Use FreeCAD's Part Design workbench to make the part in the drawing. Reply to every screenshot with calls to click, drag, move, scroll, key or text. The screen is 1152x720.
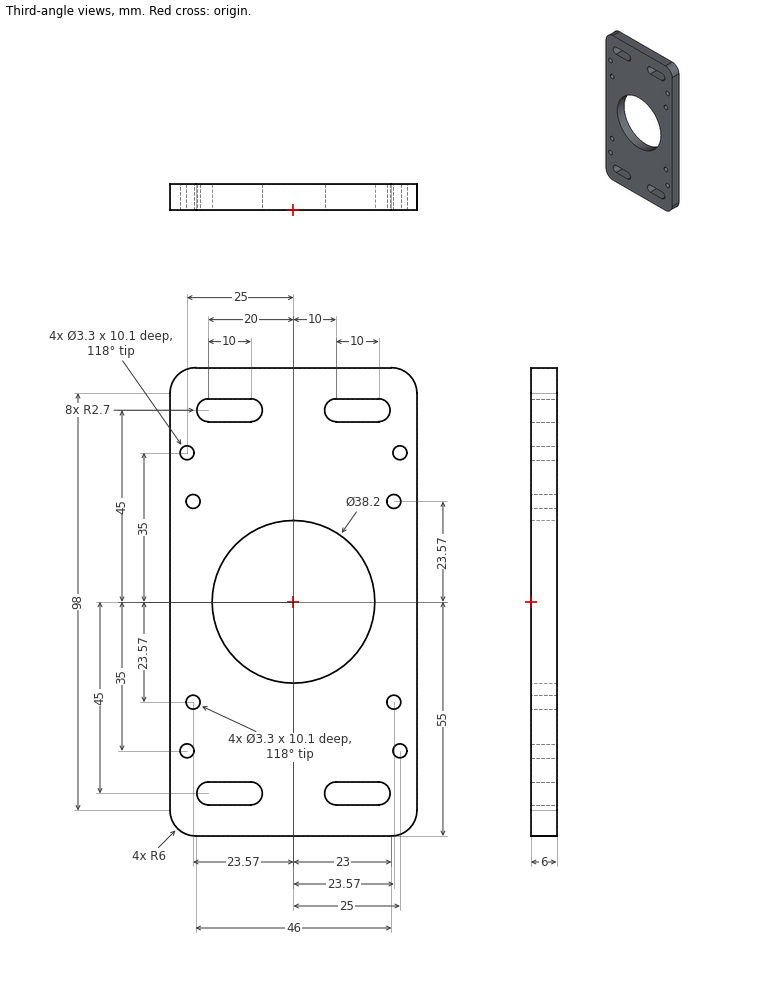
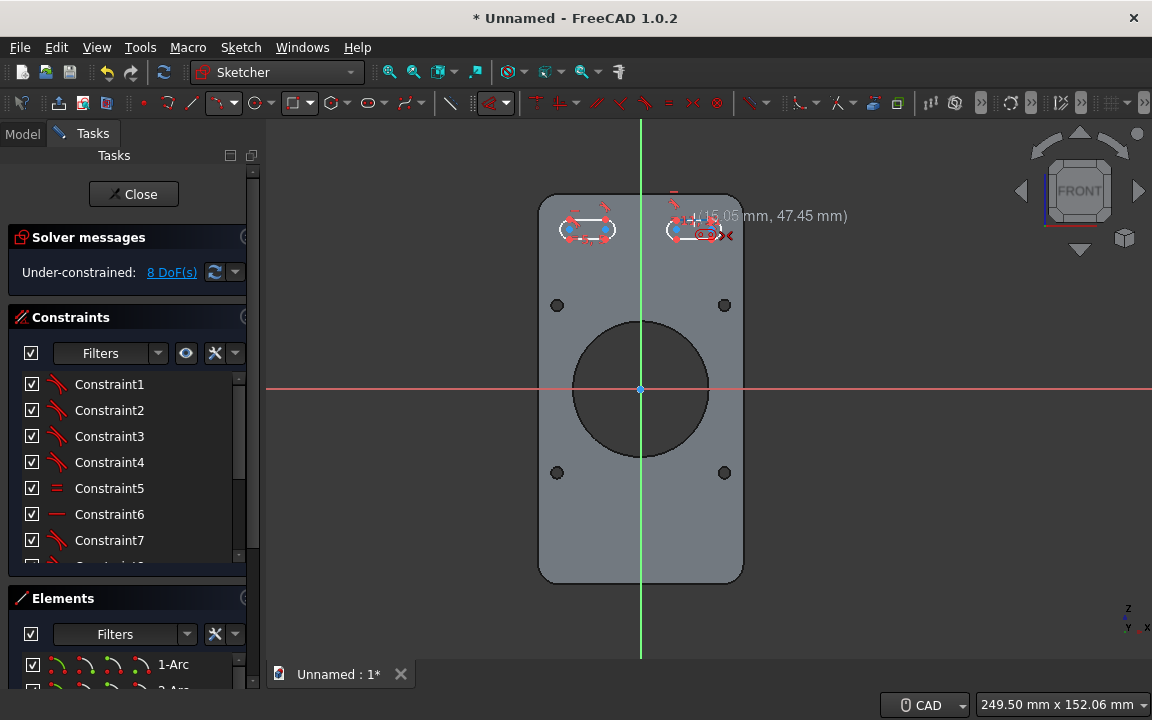
scroll(570, 549, up, 5)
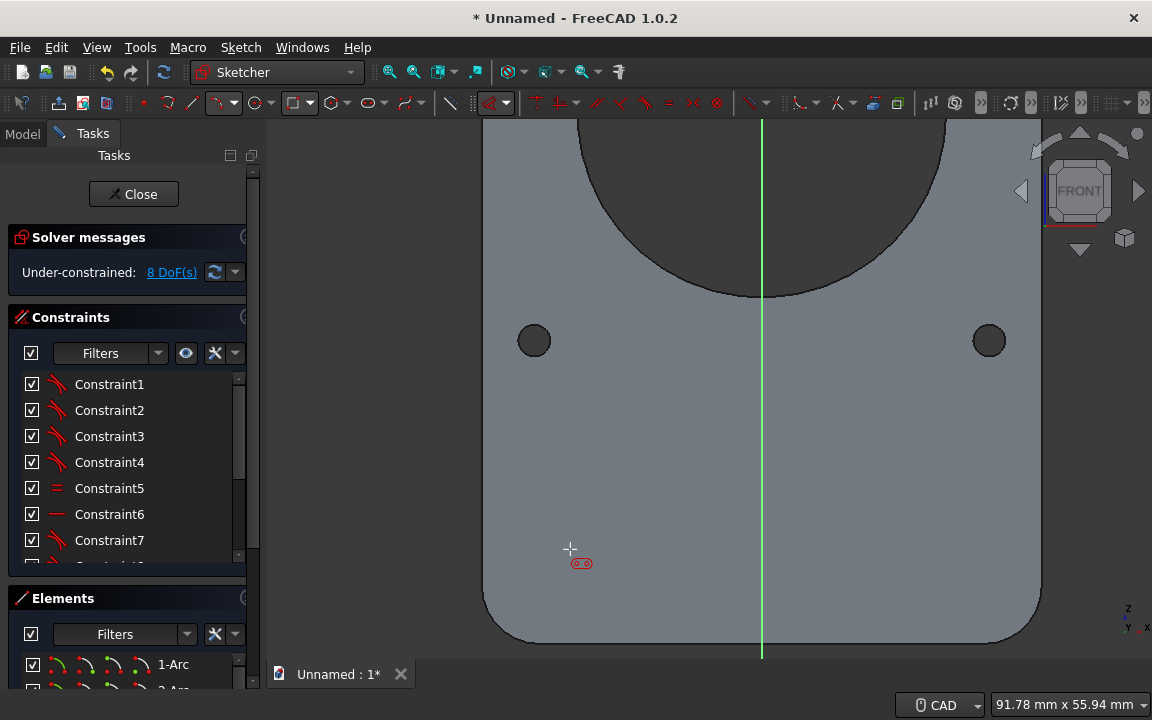
click(569, 547)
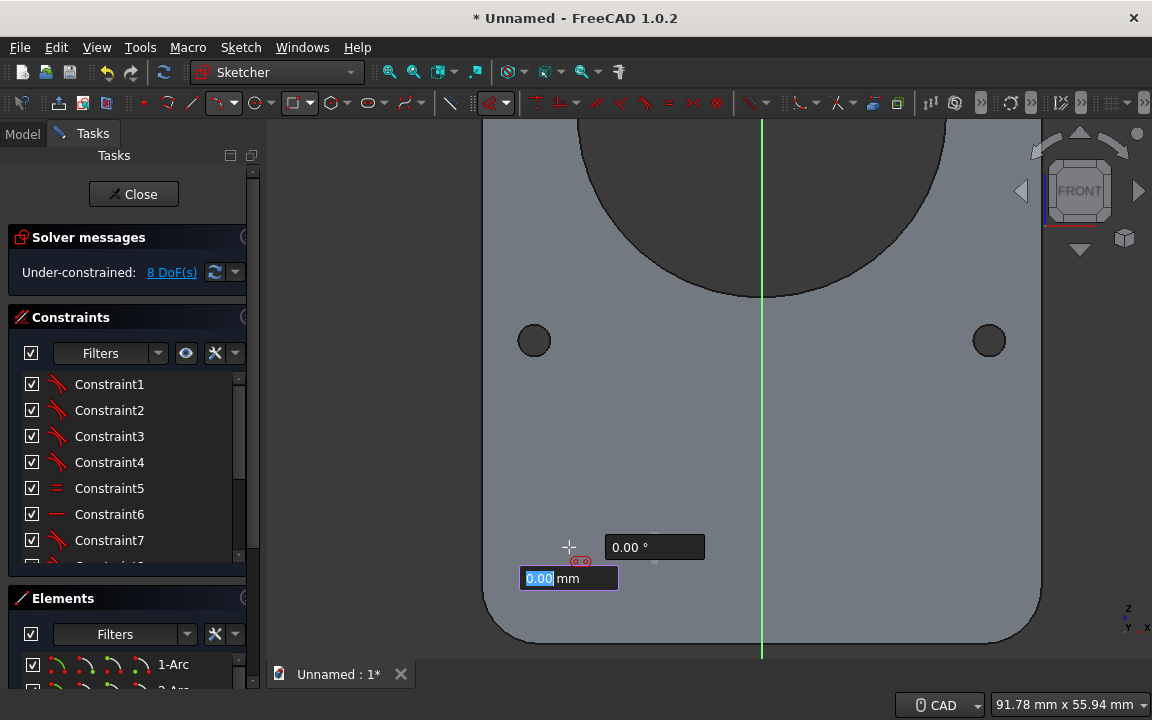
click(665, 547)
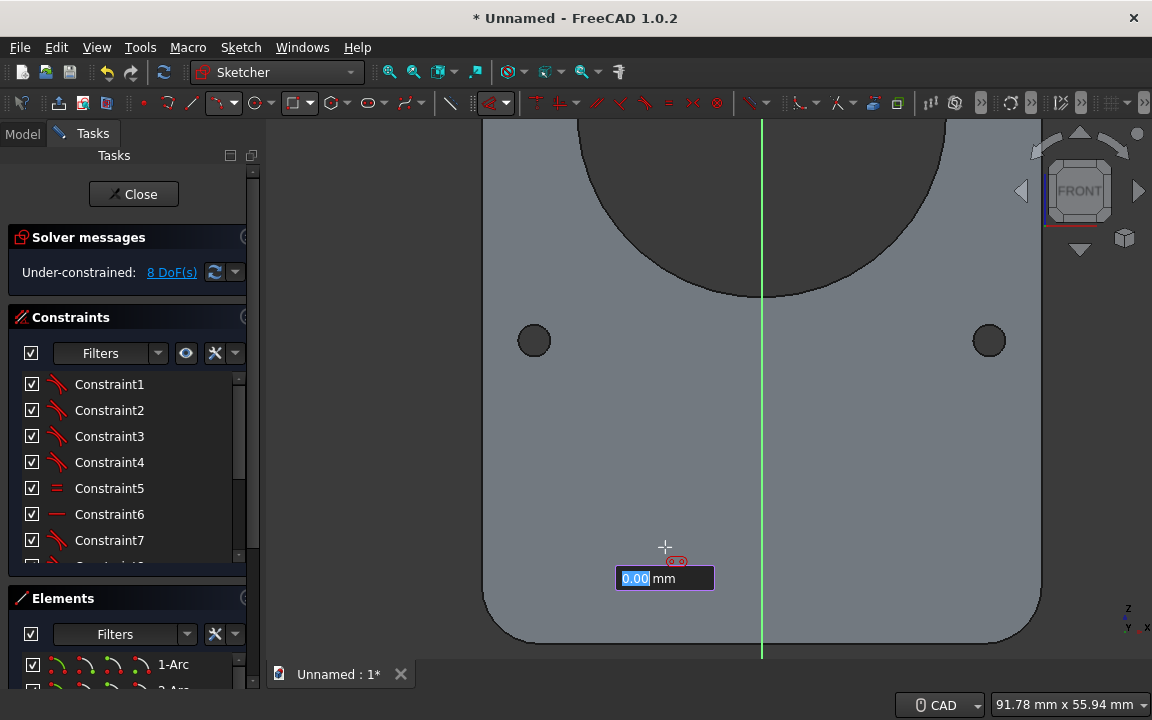
click(617, 574)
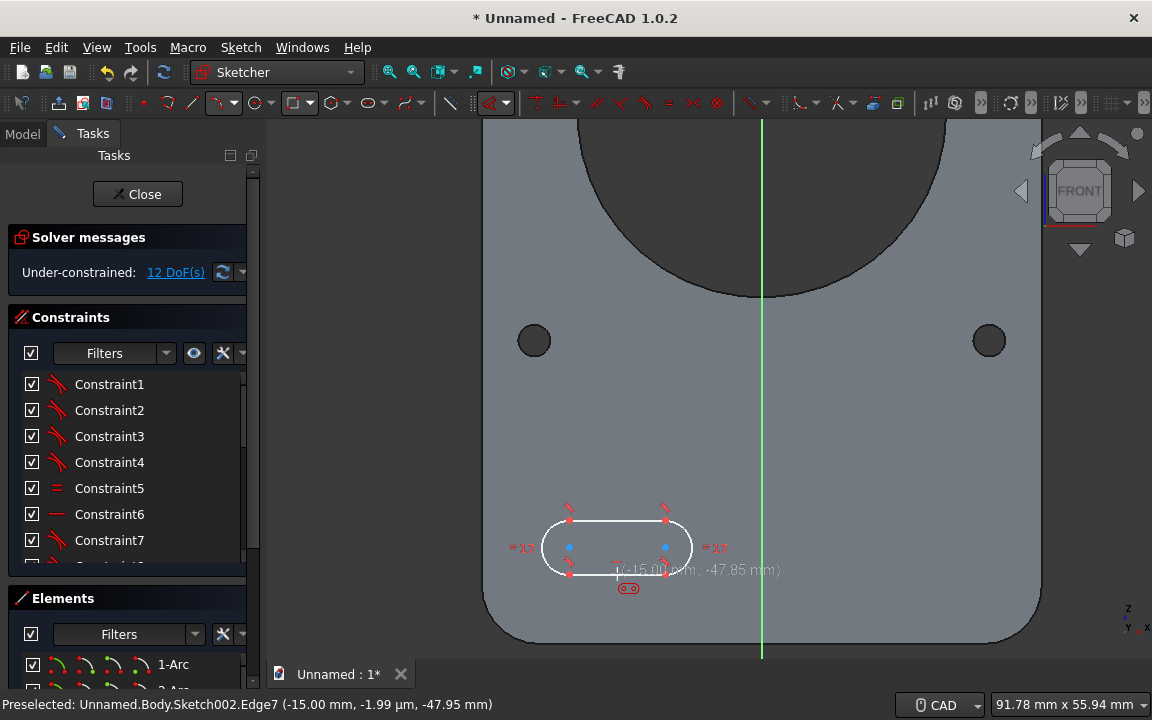
click(858, 547)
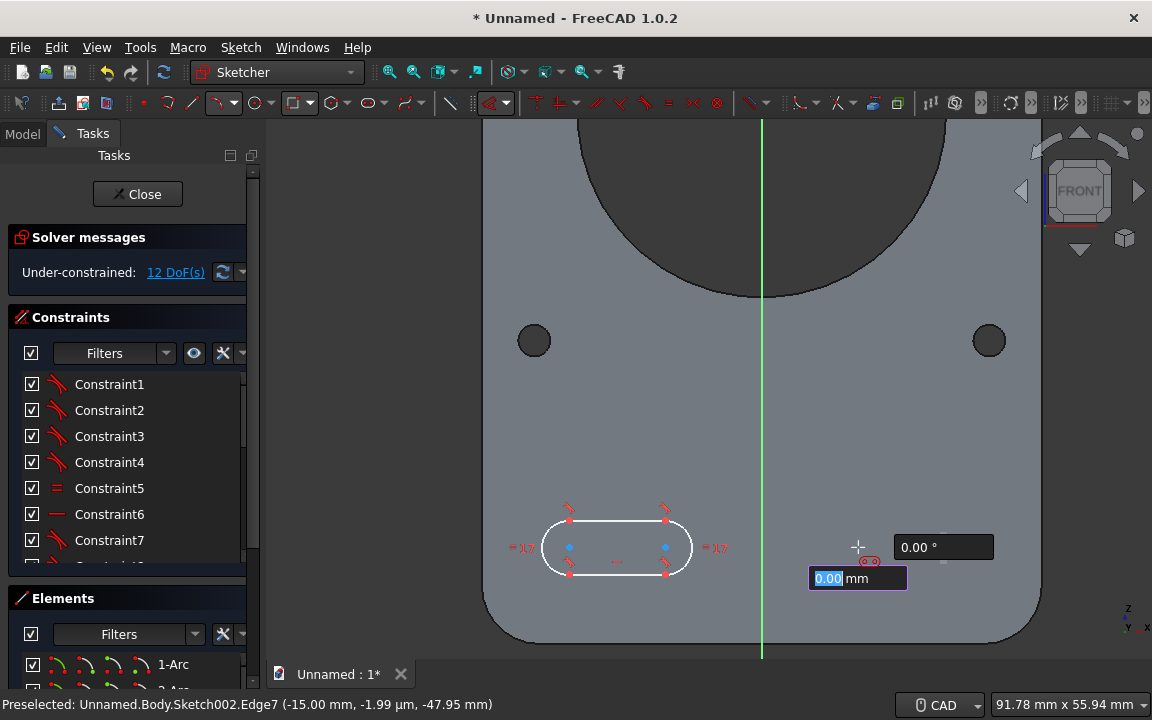
click(955, 547)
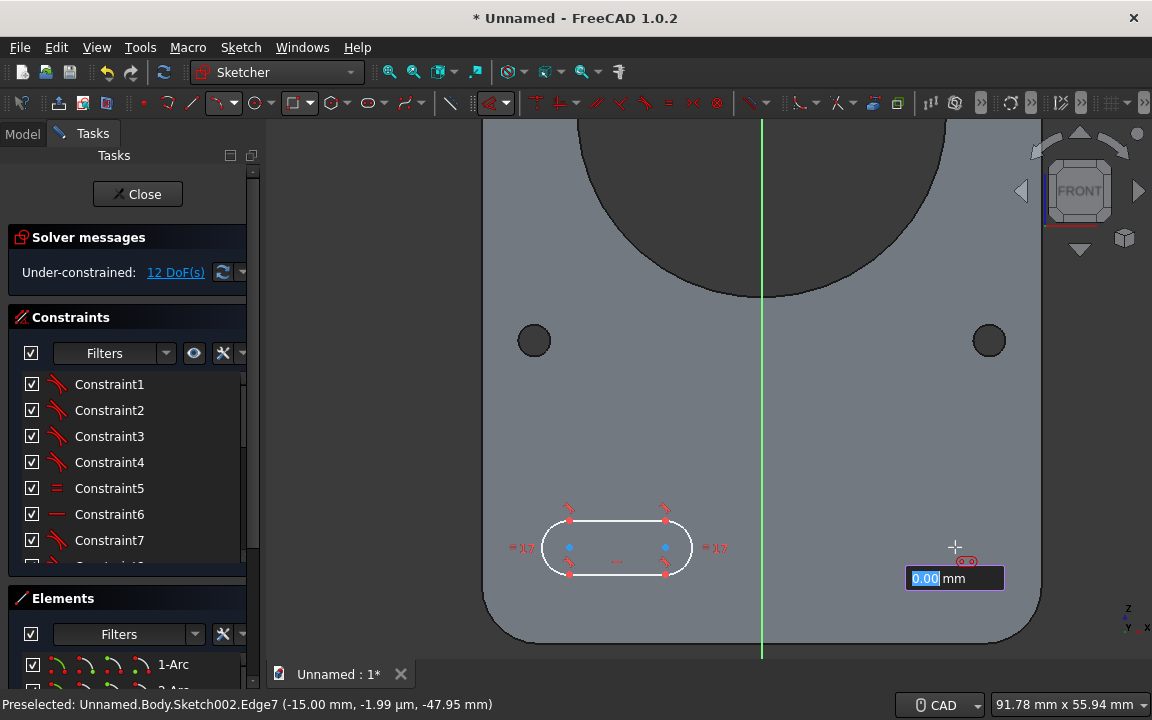
click(907, 574)
key(Escape)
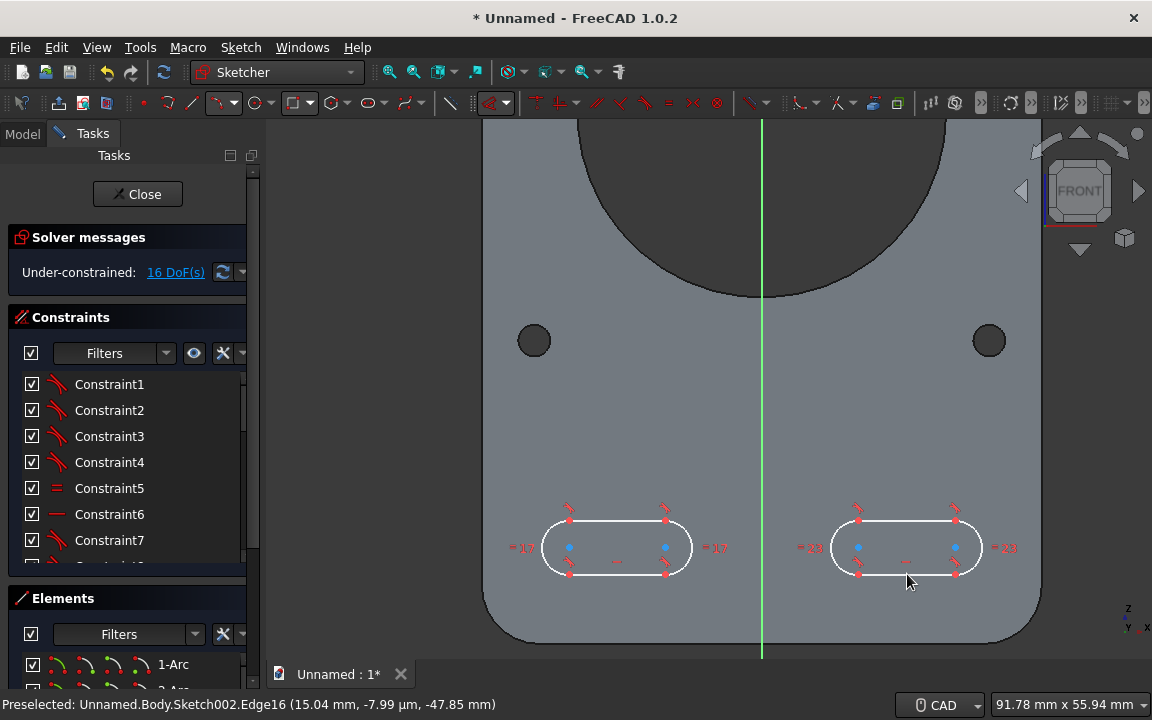
scroll(570, 550, down, 5)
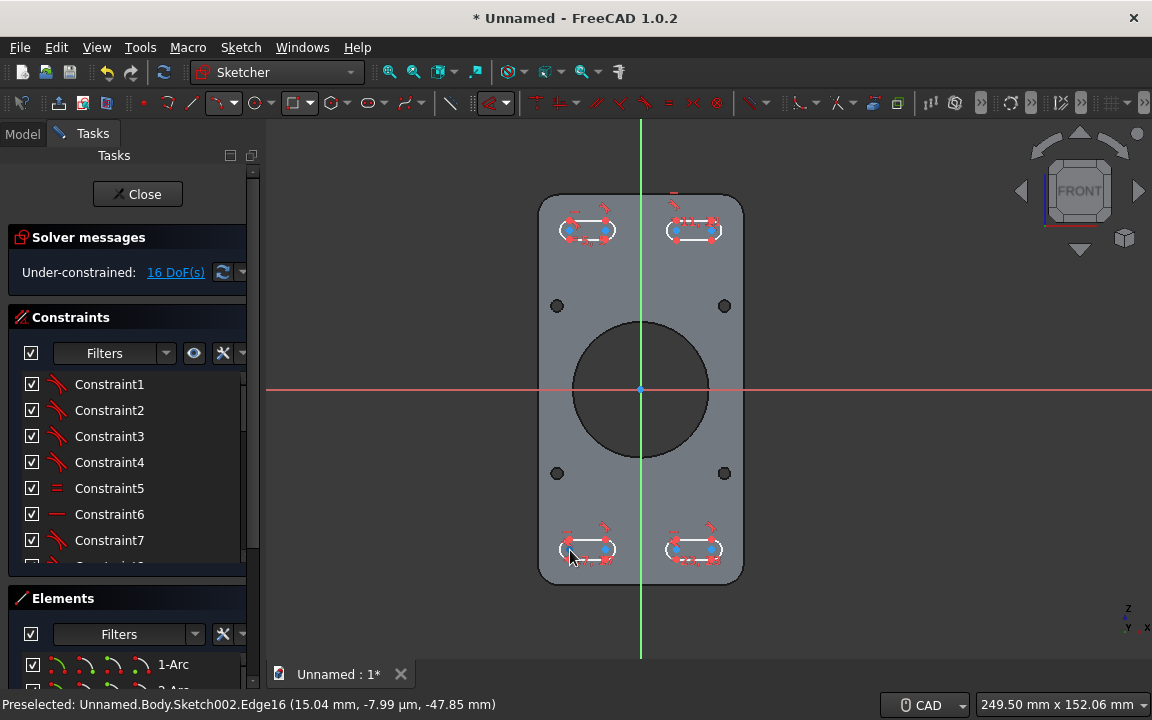
scroll(562, 225, up, 3)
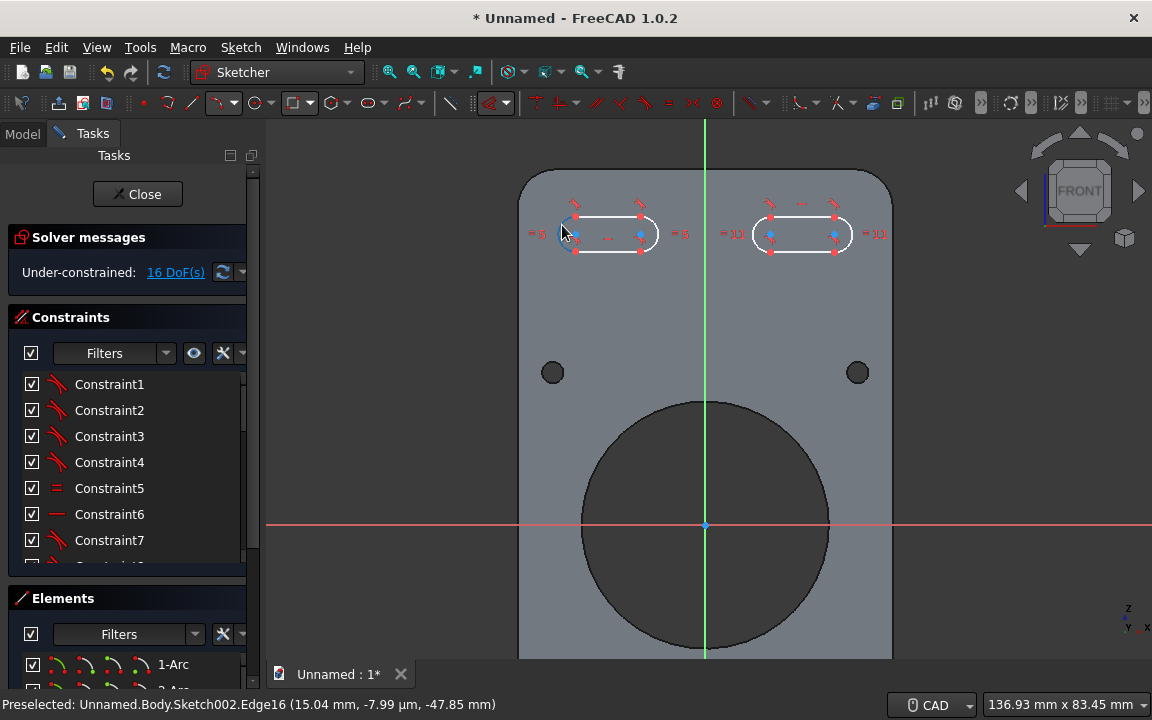
click(562, 224)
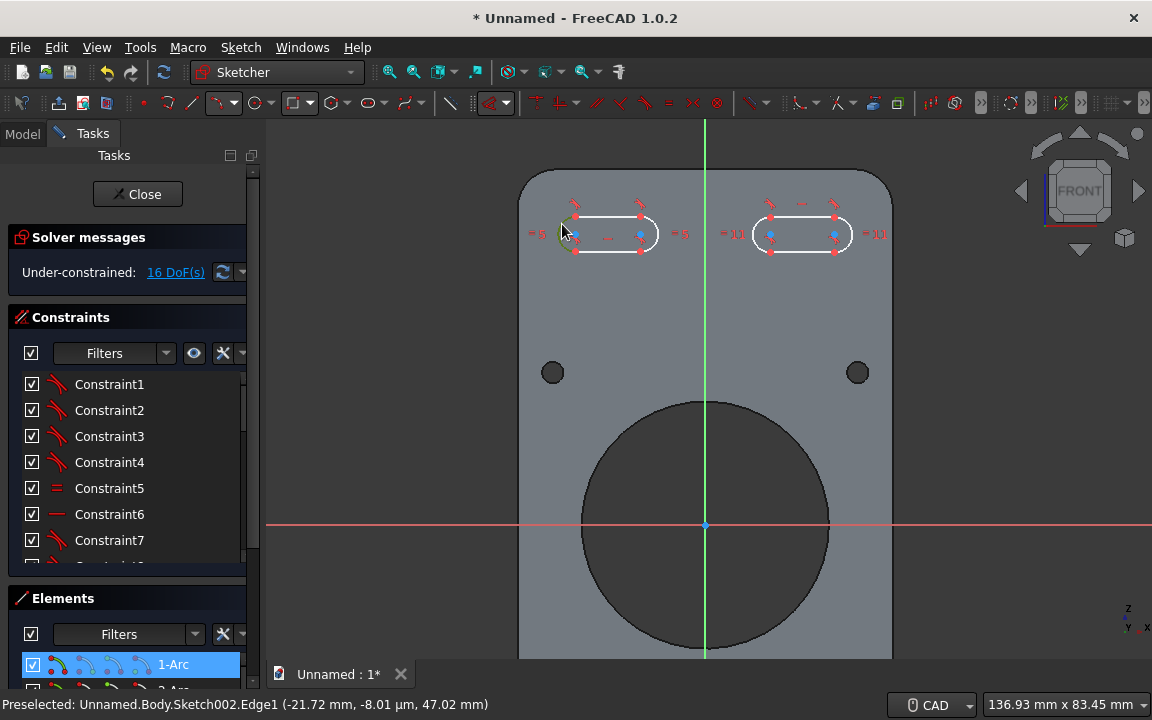
click(756, 225)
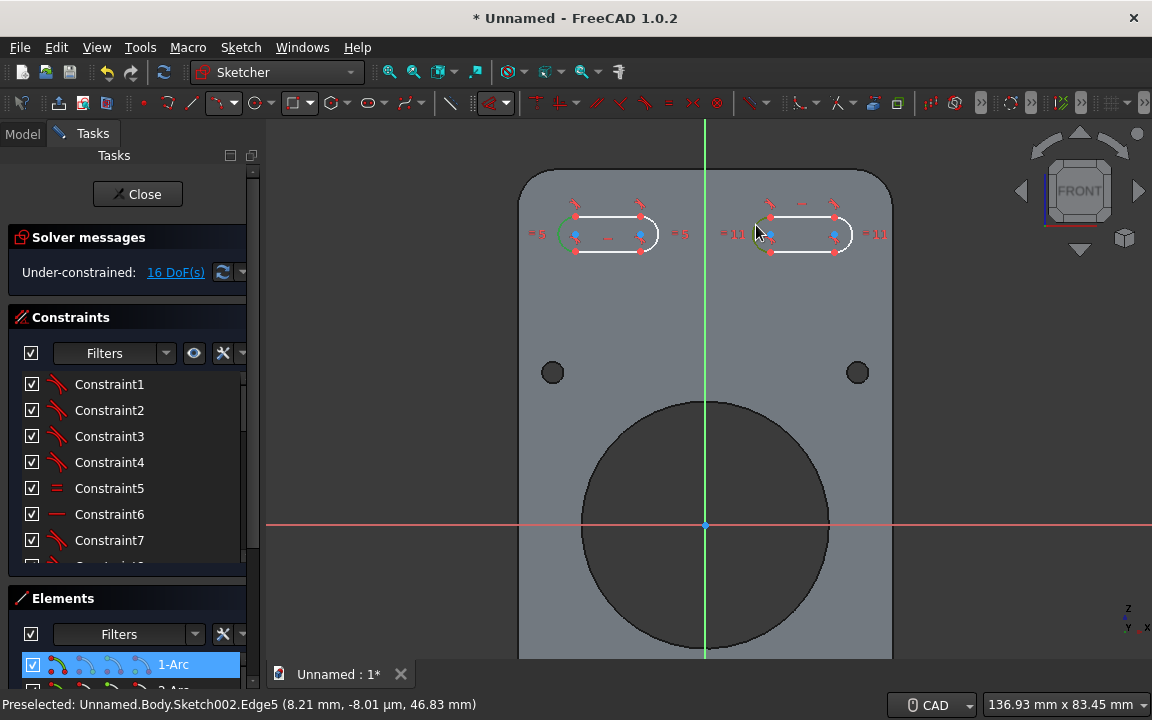
scroll(562, 223, down, 3)